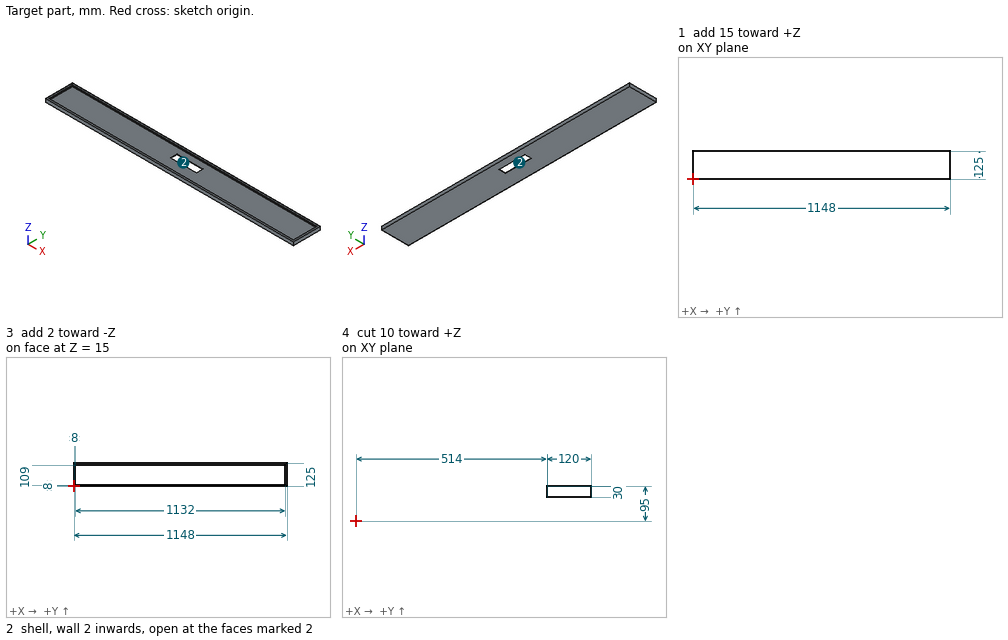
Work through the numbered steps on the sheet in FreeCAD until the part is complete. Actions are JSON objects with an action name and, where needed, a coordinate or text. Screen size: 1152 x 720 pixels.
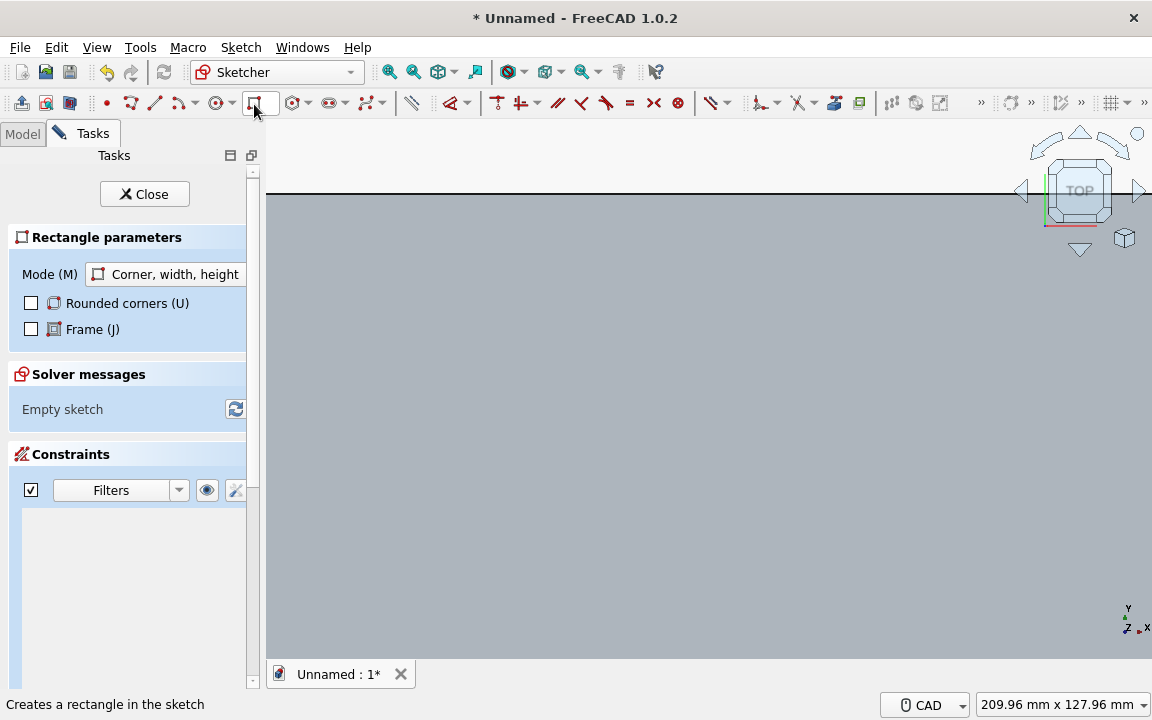
{"action": "left_click", "coordinate": [379, 320]}
{"action": "mouse_move", "coordinate": [886, 447]}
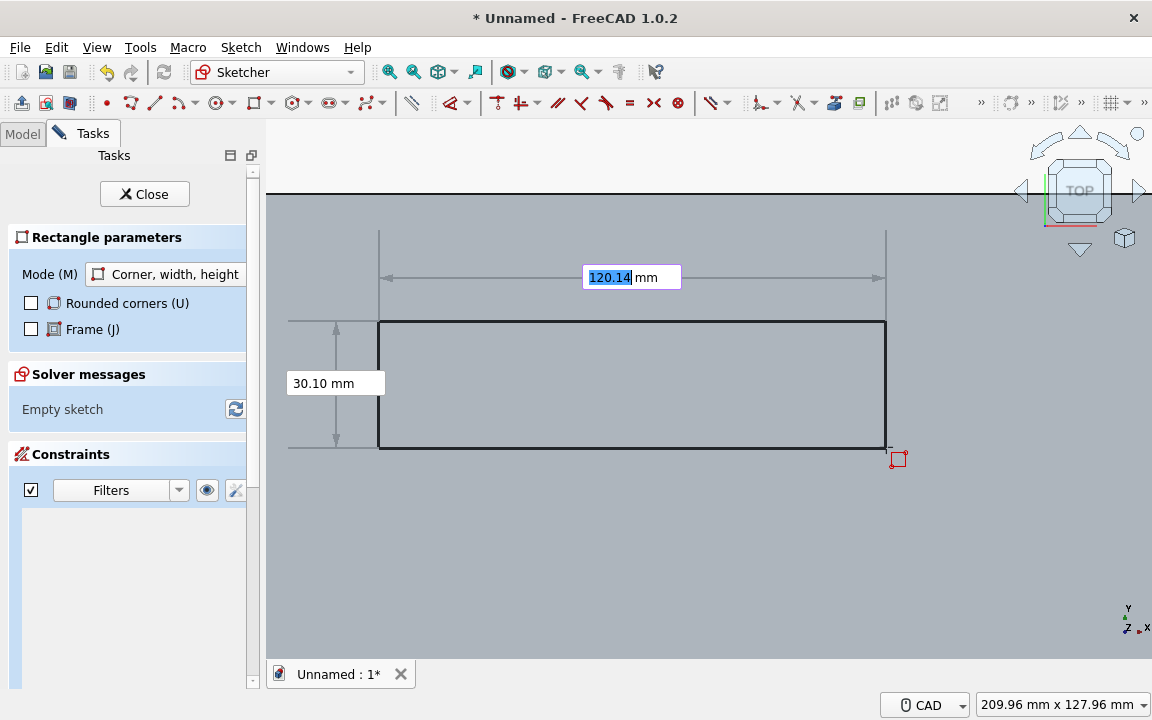
{"action": "type", "text": "120"}
{"action": "key", "text": "Tab"}
{"action": "type", "text": "30"}
{"action": "key", "text": "Return"}
{"action": "key", "text": "Escape"}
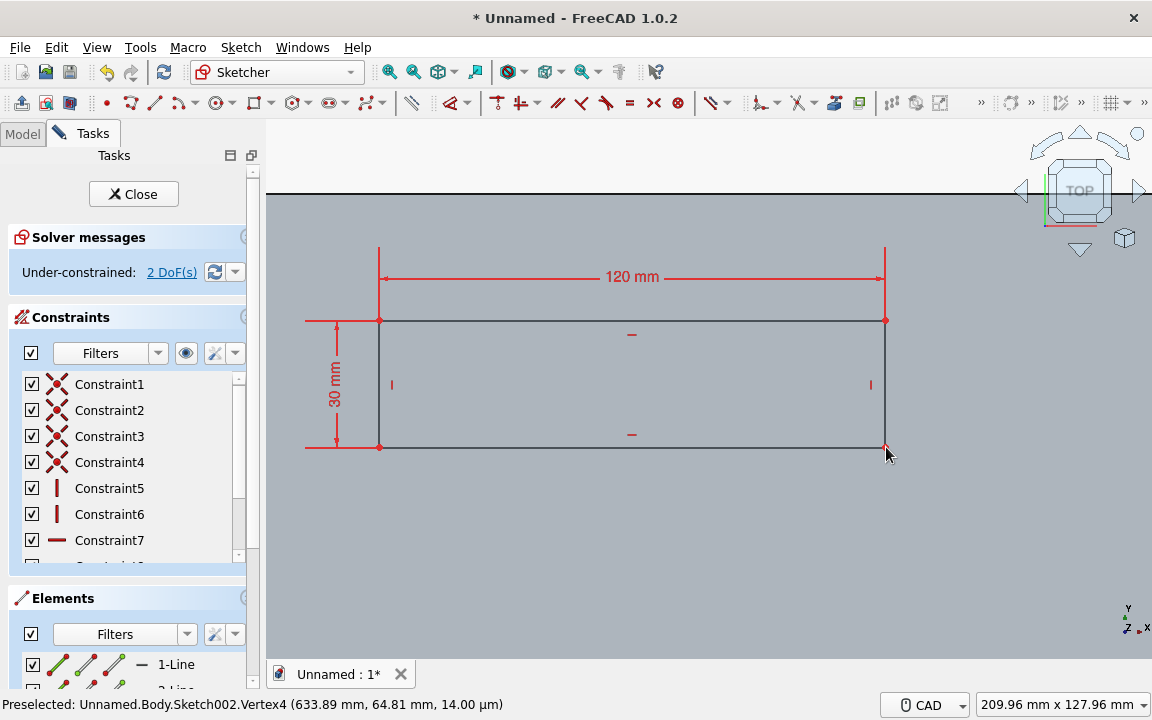
{"action": "left_click", "coordinate": [450, 104]}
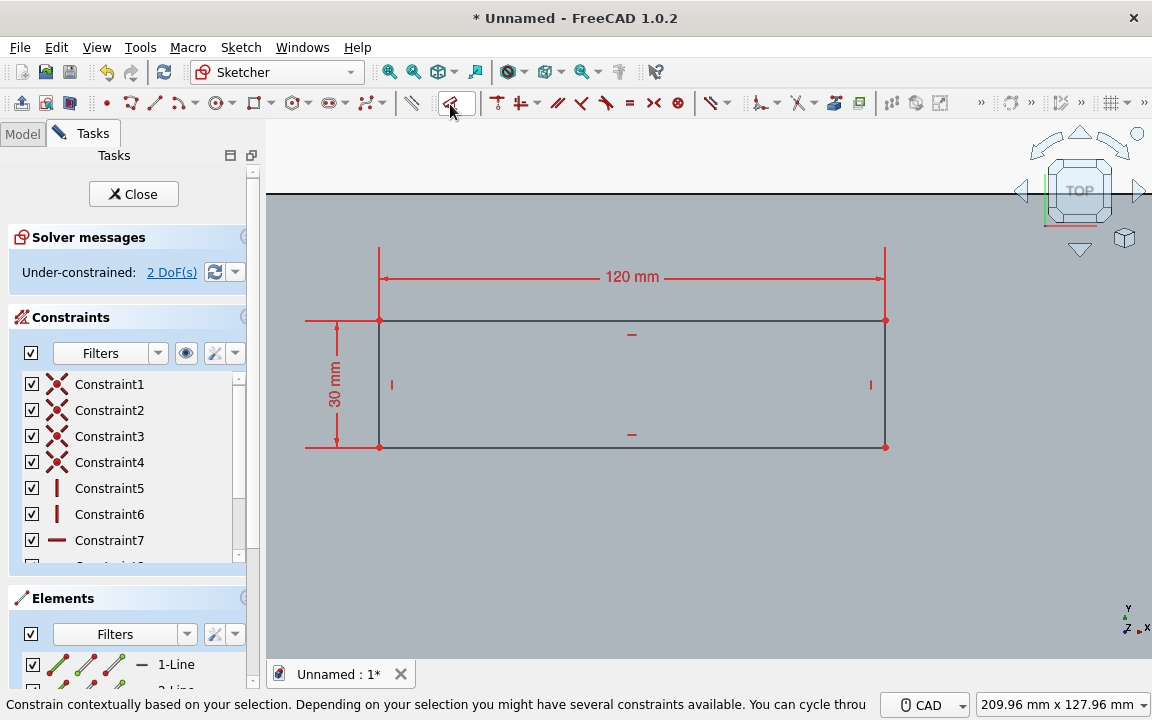
{"action": "left_click", "coordinate": [379, 321]}
{"action": "left_click", "coordinate": [413, 476]}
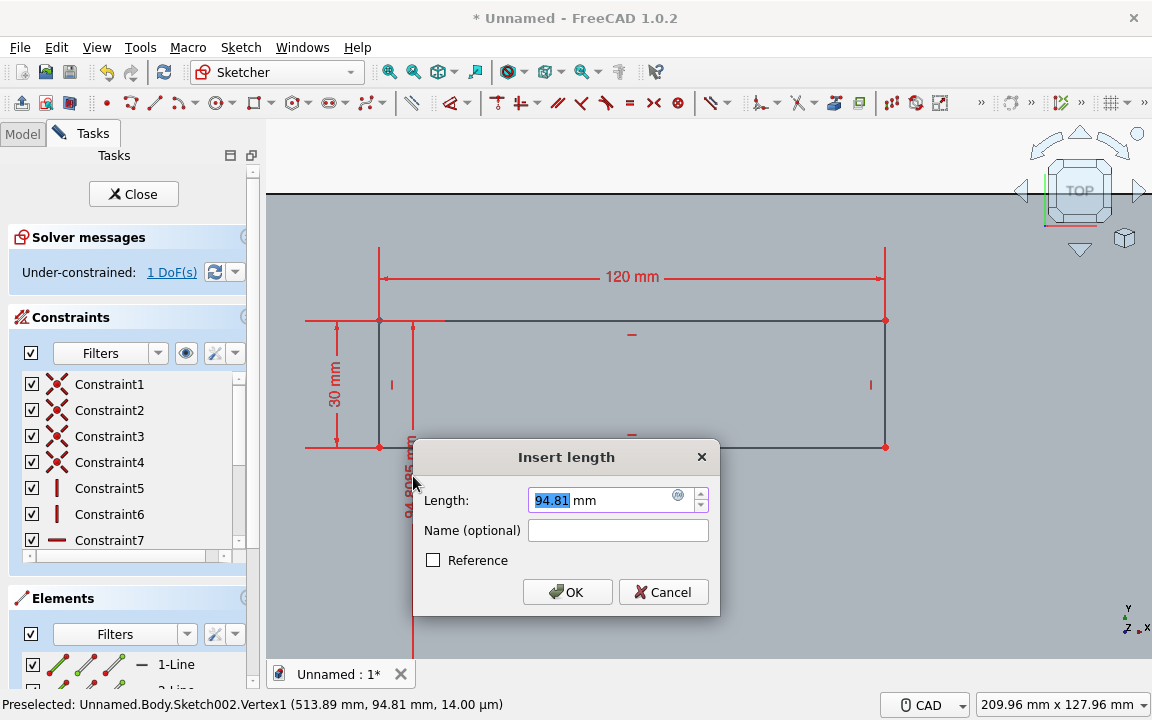
{"action": "type", "text": "95"}
{"action": "key", "text": "Return"}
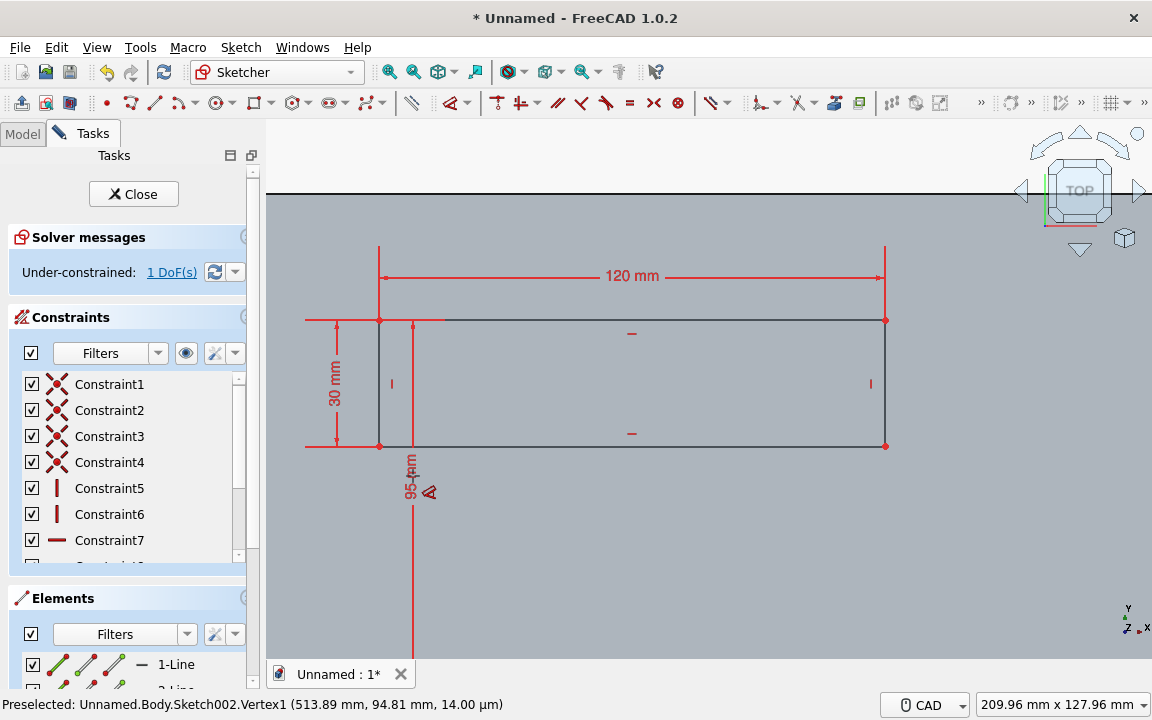
{"action": "left_click", "coordinate": [379, 320]}
{"action": "left_click", "coordinate": [337, 286]}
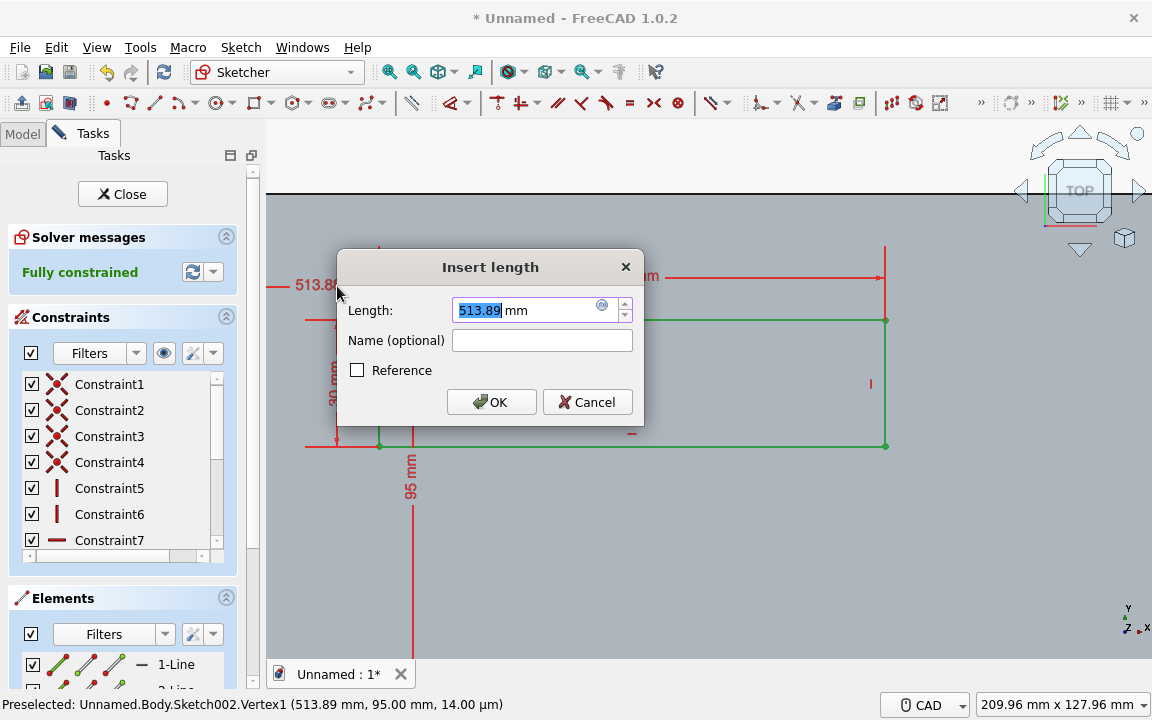
{"action": "type", "text": "514"}
{"action": "key", "text": "Return"}
{"action": "key", "text": "Escape"}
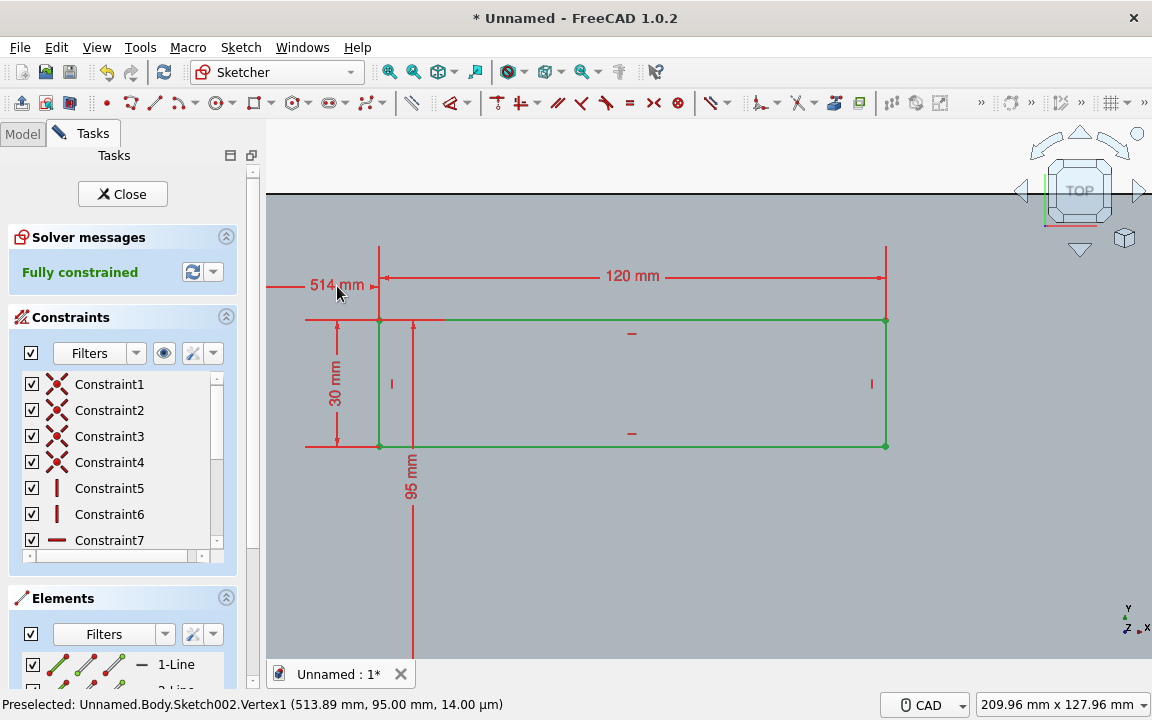
{"action": "left_click", "coordinate": [123, 194]}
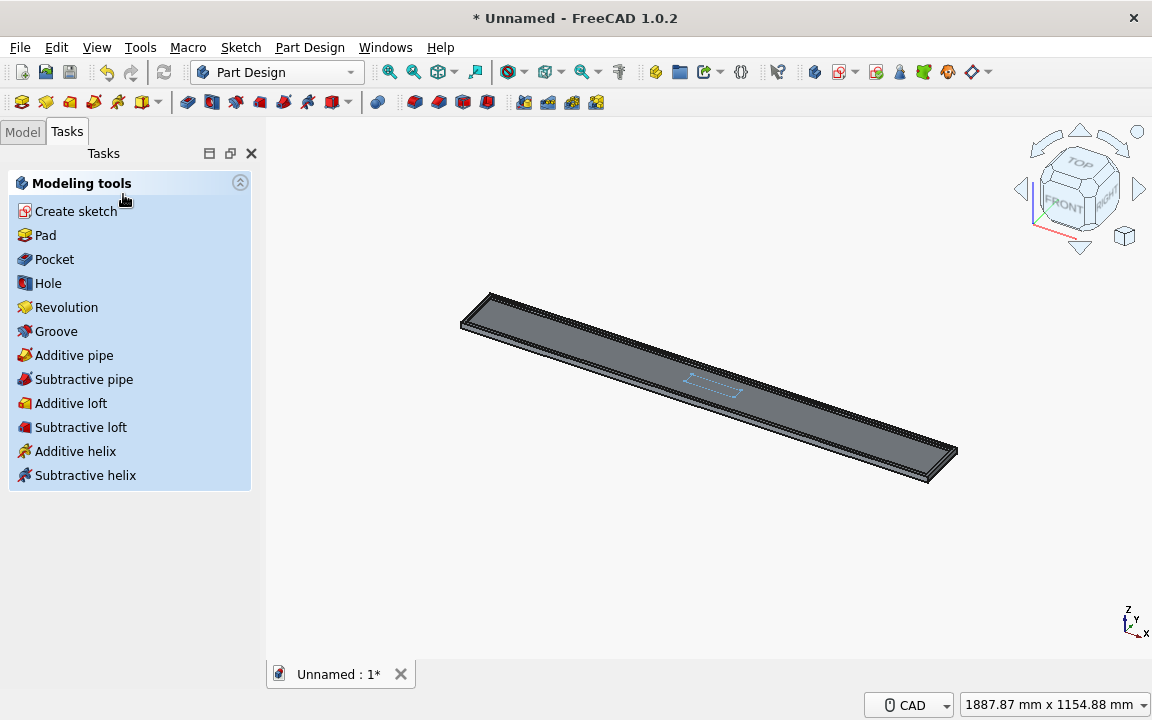
{"action": "left_click", "coordinate": [188, 102]}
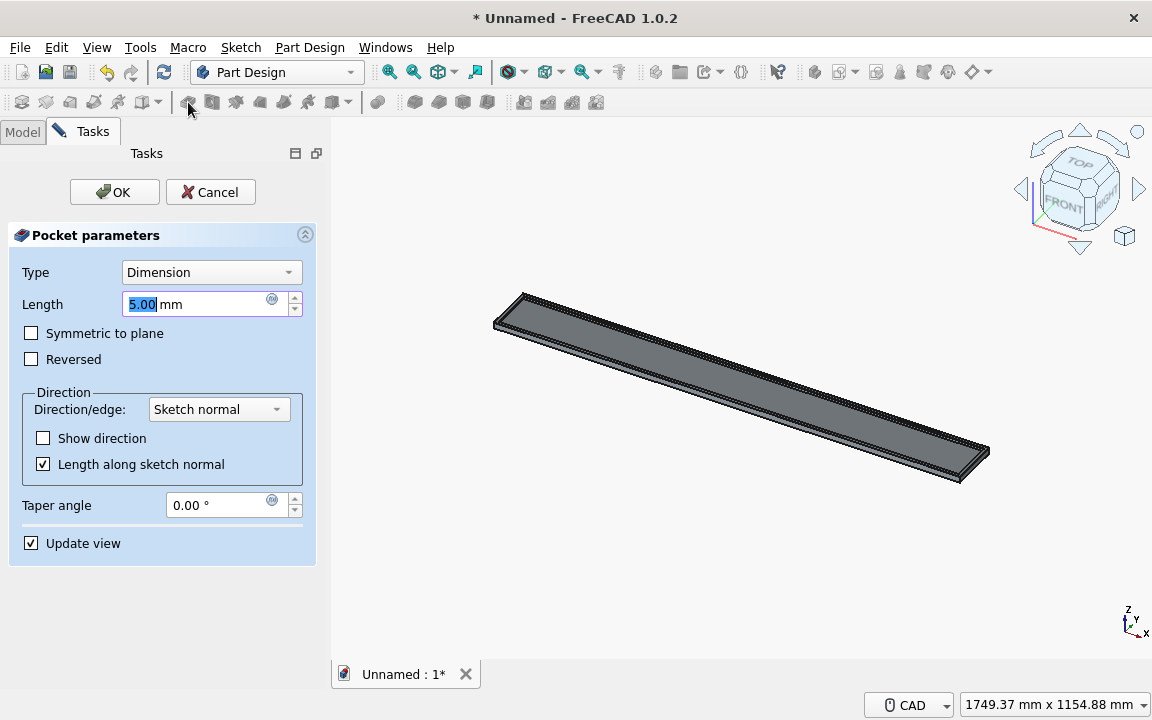
{"action": "type", "text": "10"}
{"action": "key", "text": "Tab"}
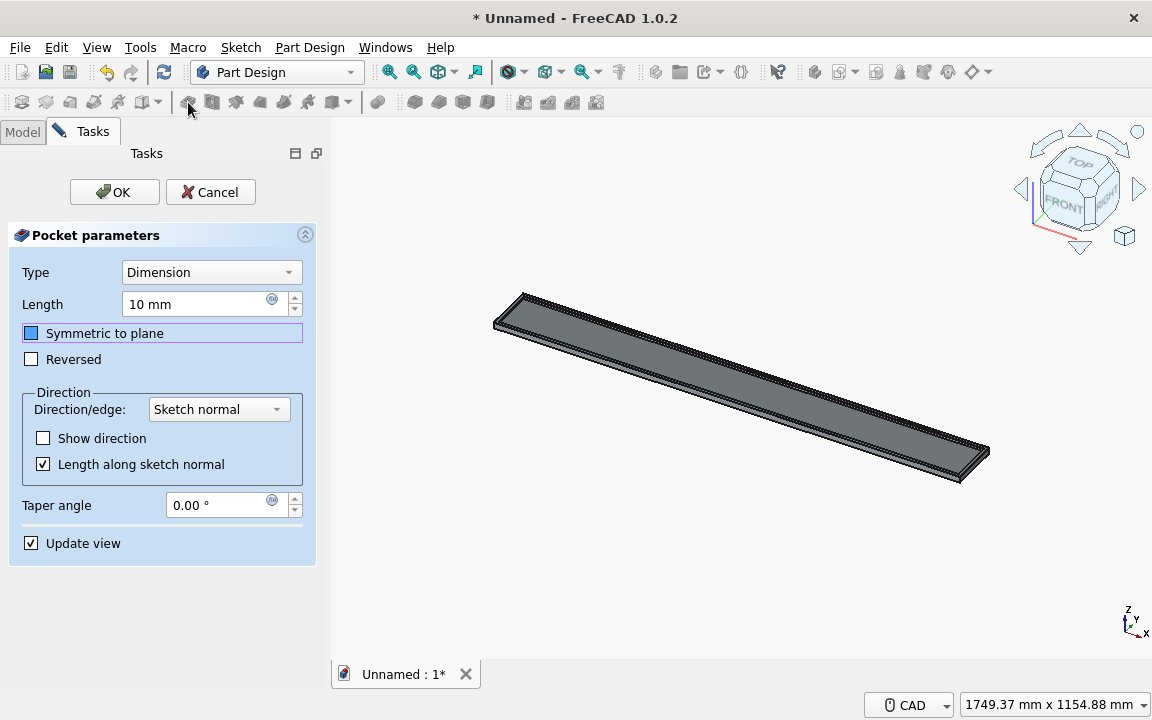
{"action": "left_click", "coordinate": [30, 359]}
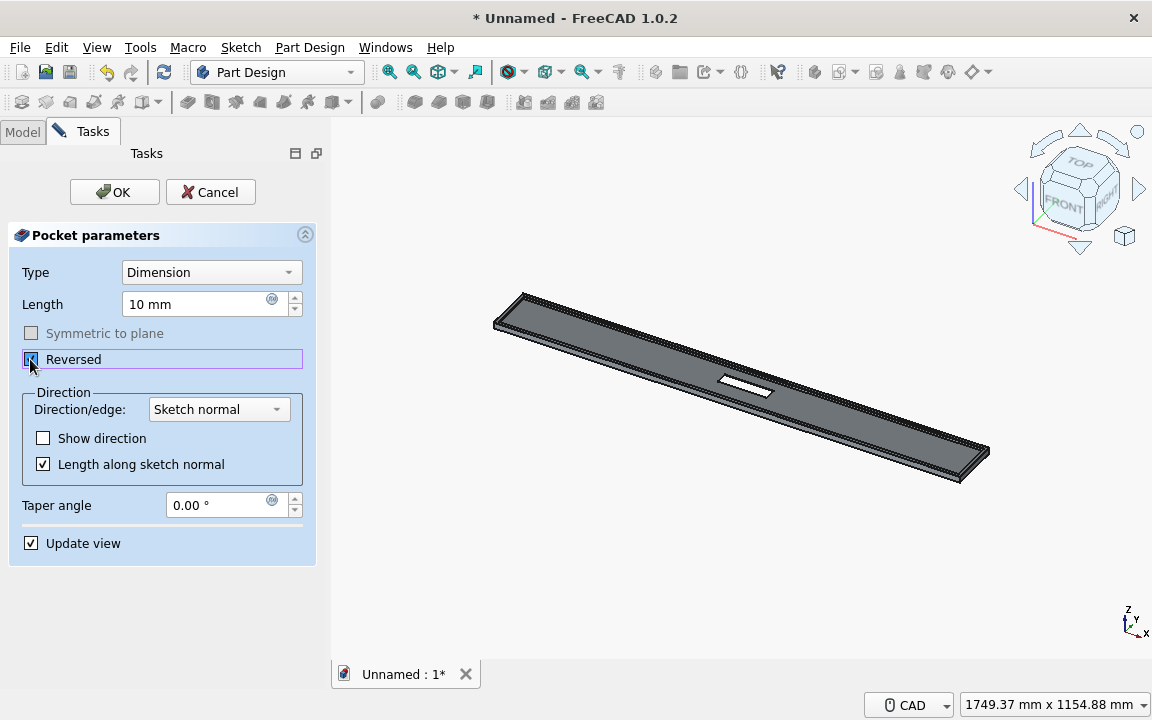
{"action": "left_click", "coordinate": [115, 192]}